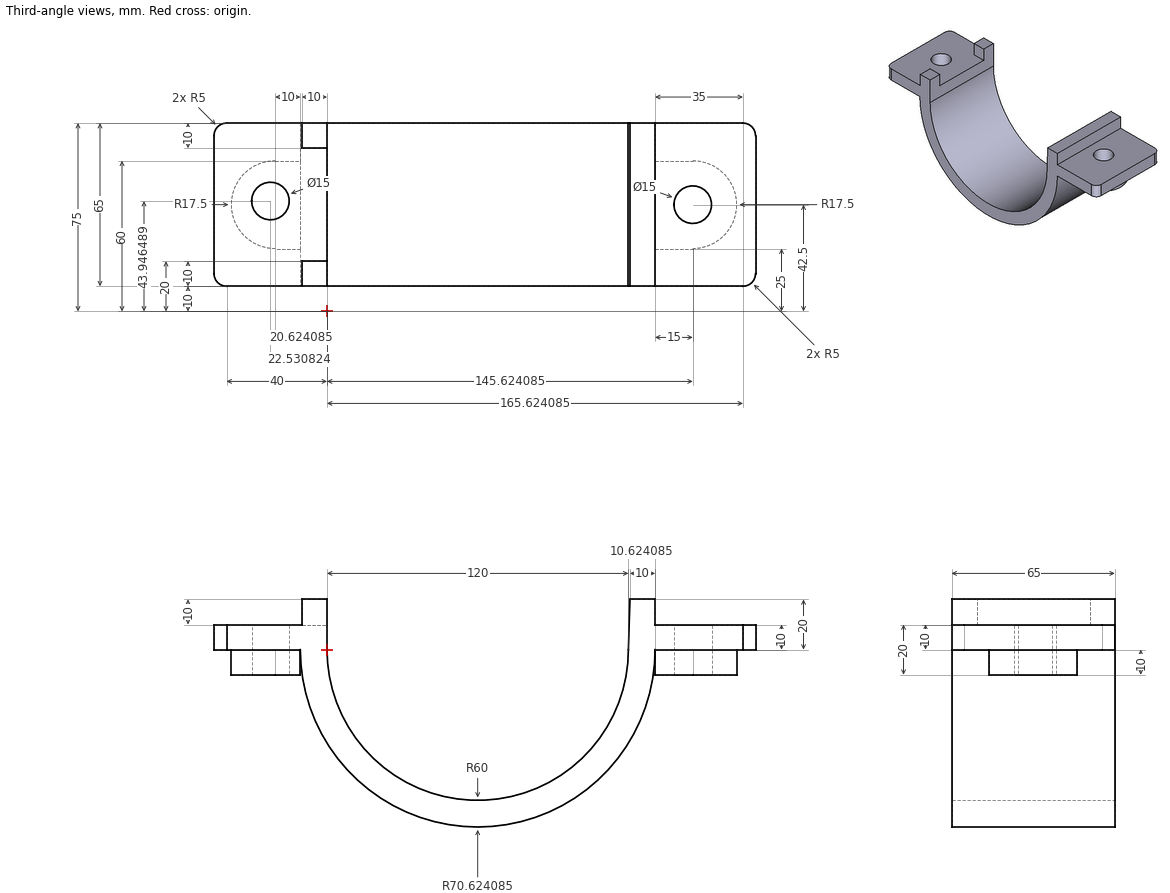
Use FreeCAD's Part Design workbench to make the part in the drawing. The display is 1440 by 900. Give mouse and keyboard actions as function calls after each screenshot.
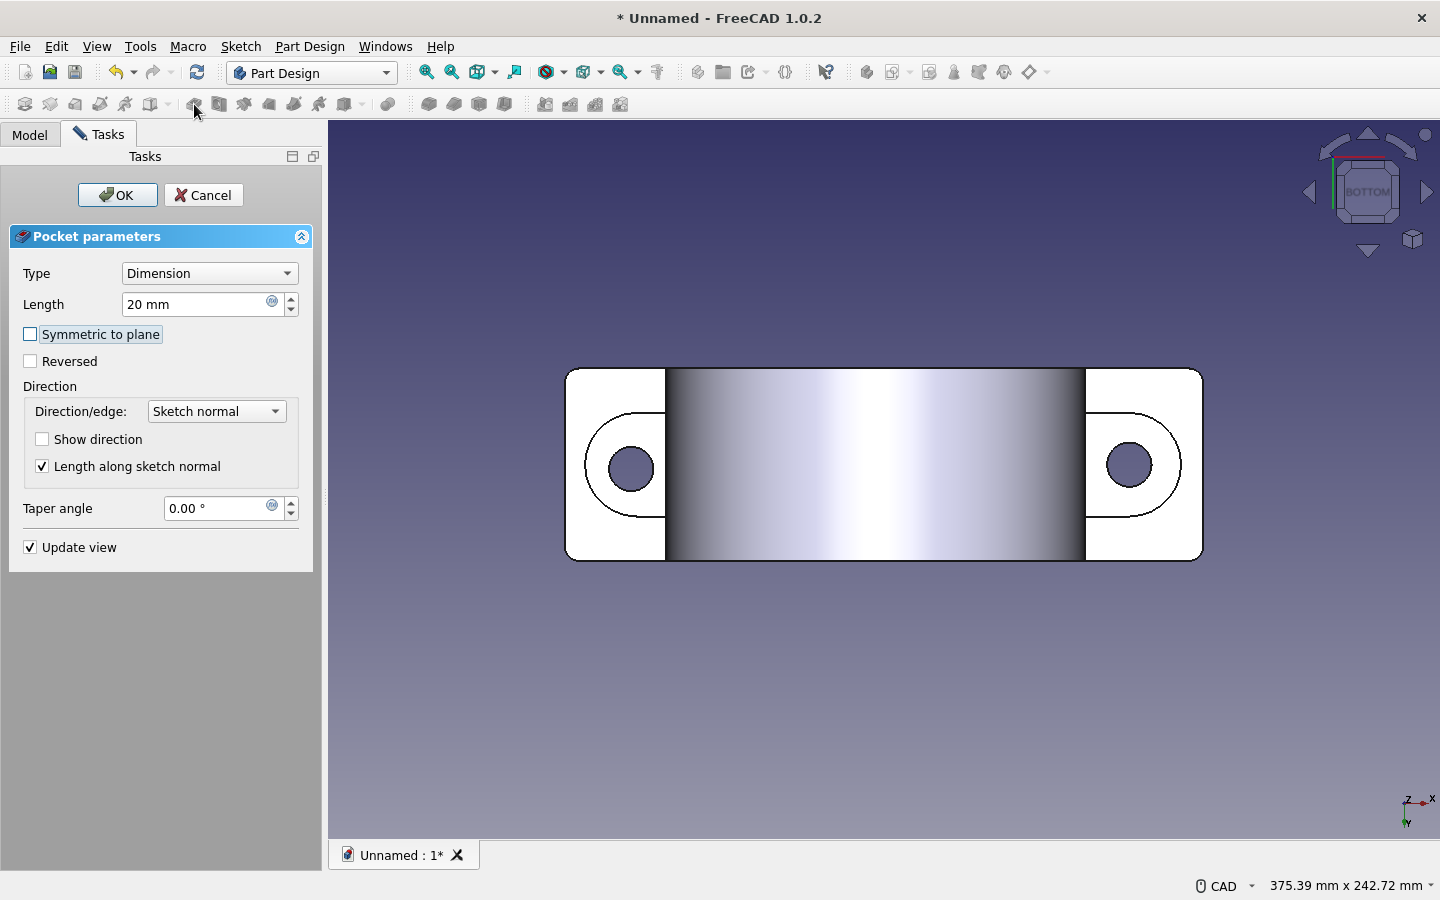
click(118, 195)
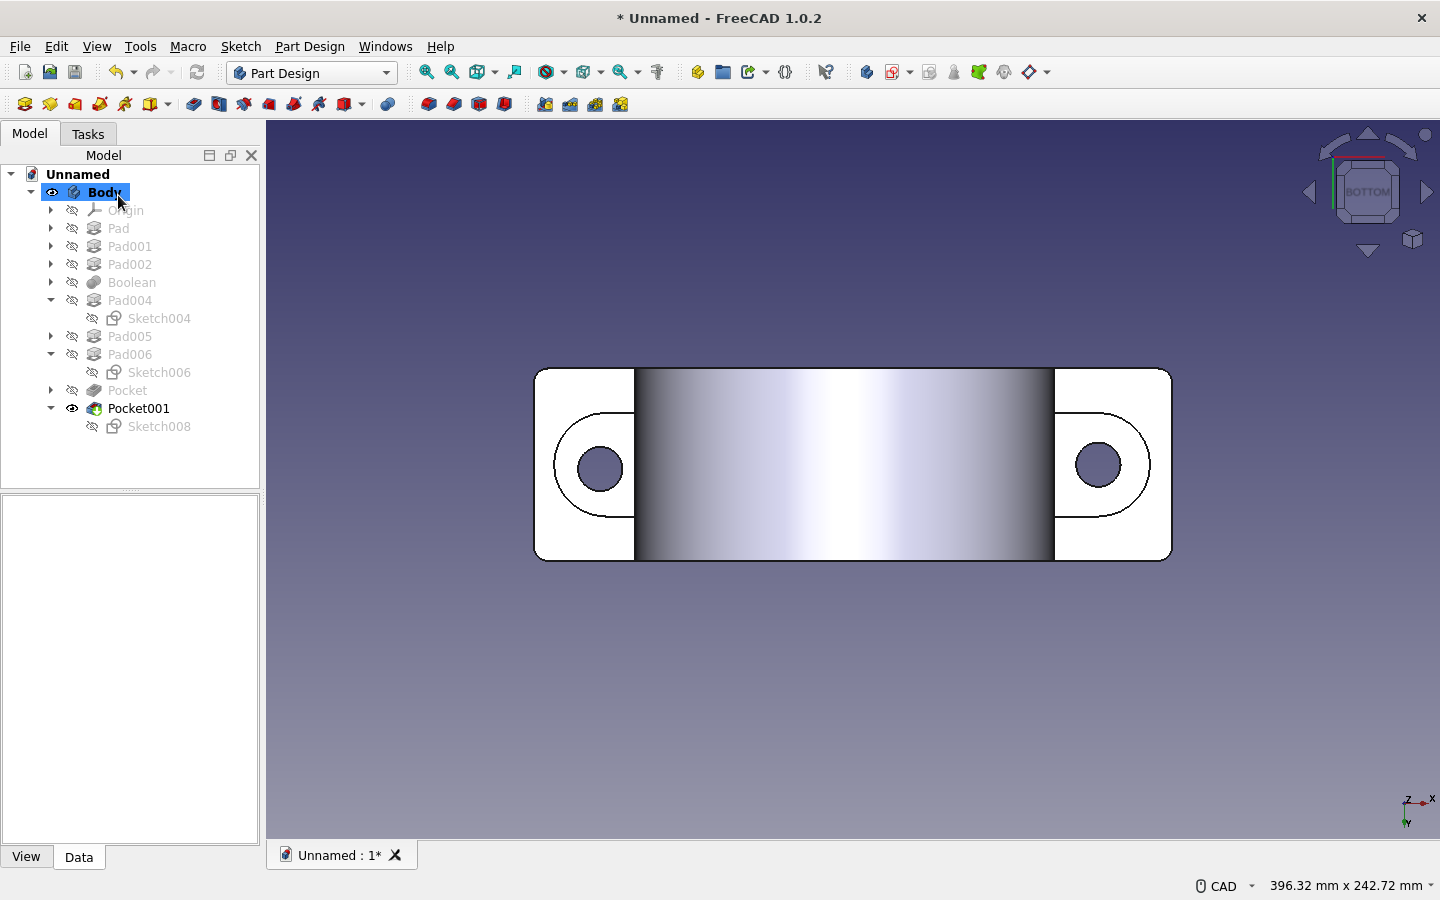
key(0)